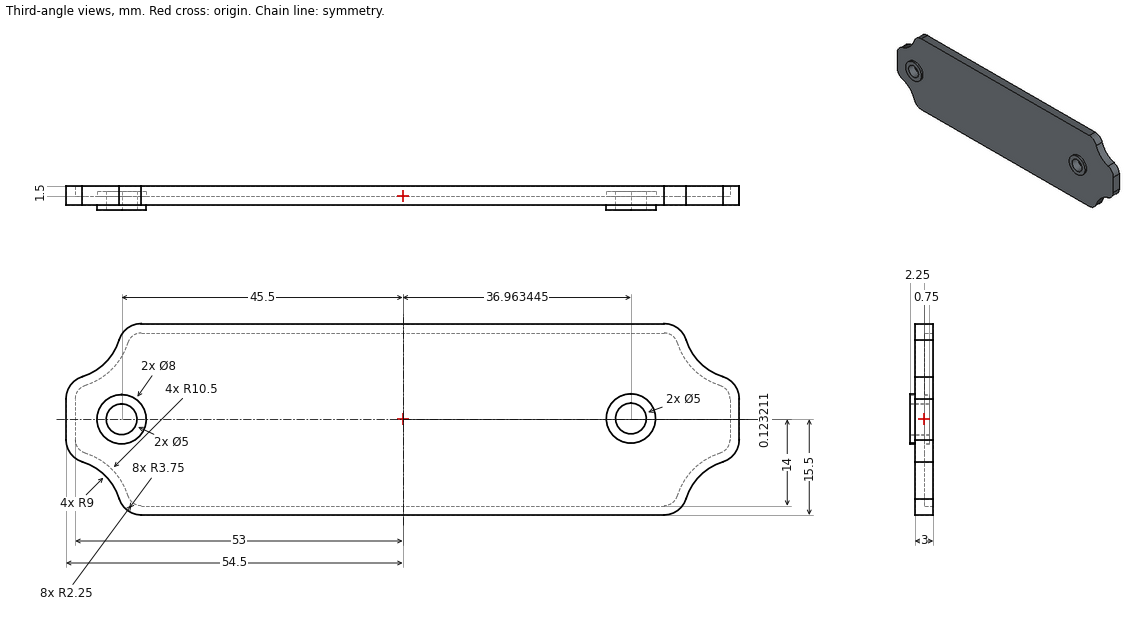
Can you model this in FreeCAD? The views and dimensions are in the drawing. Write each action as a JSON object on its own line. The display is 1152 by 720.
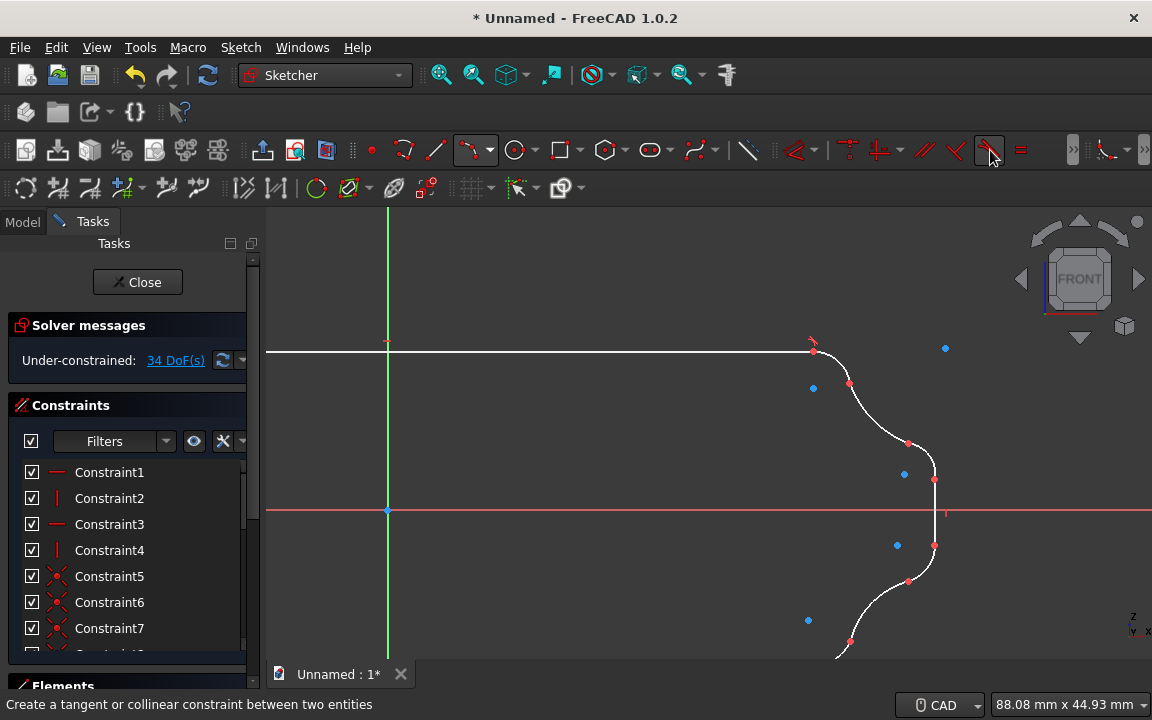
{"action": "scroll", "coordinate": [935, 499], "scroll_direction": "up", "scroll_amount": 2}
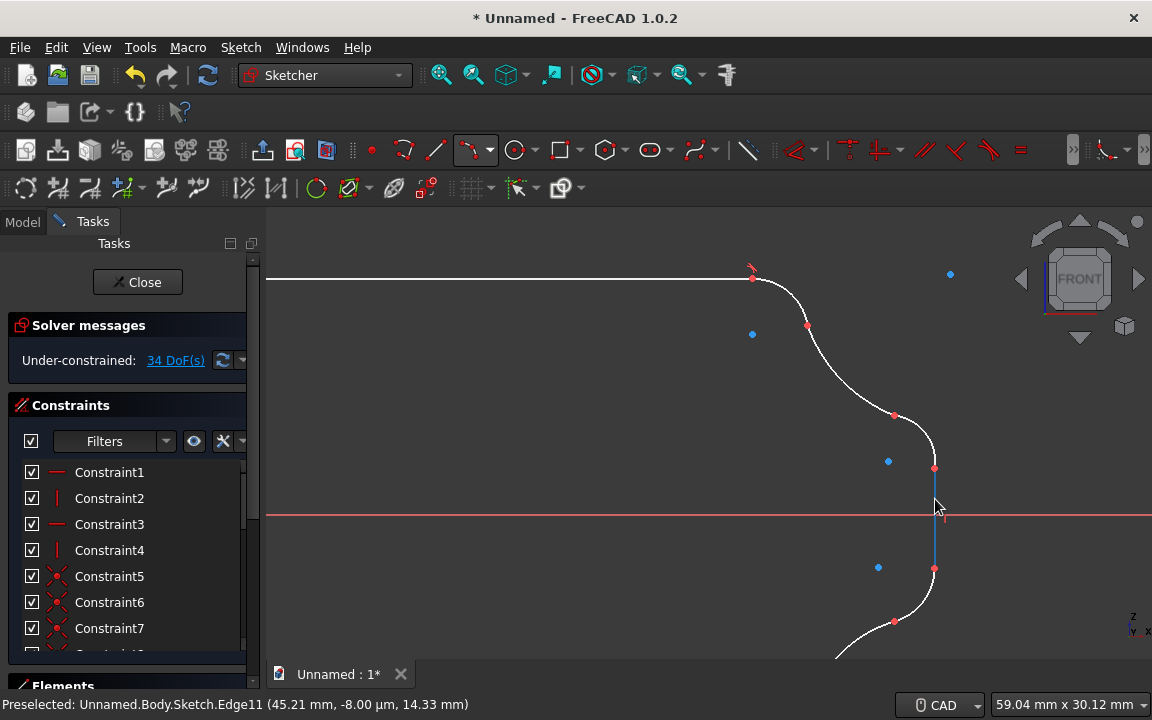
{"action": "left_click", "coordinate": [935, 499]}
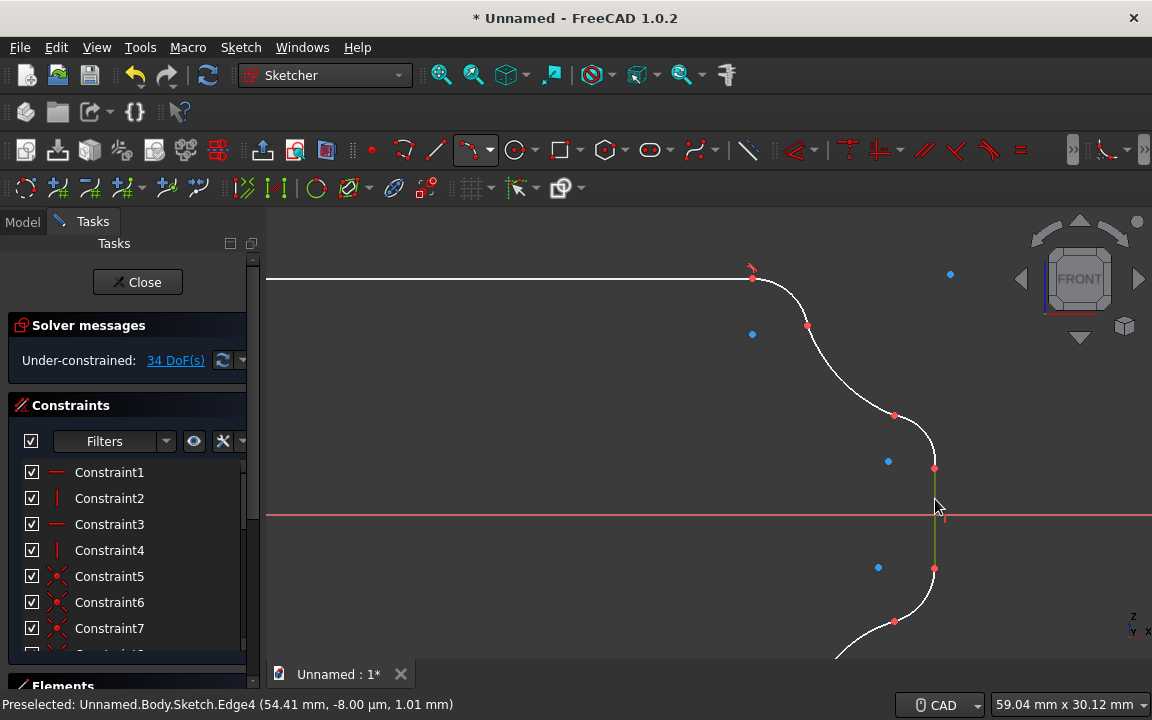
{"action": "left_click", "coordinate": [933, 447]}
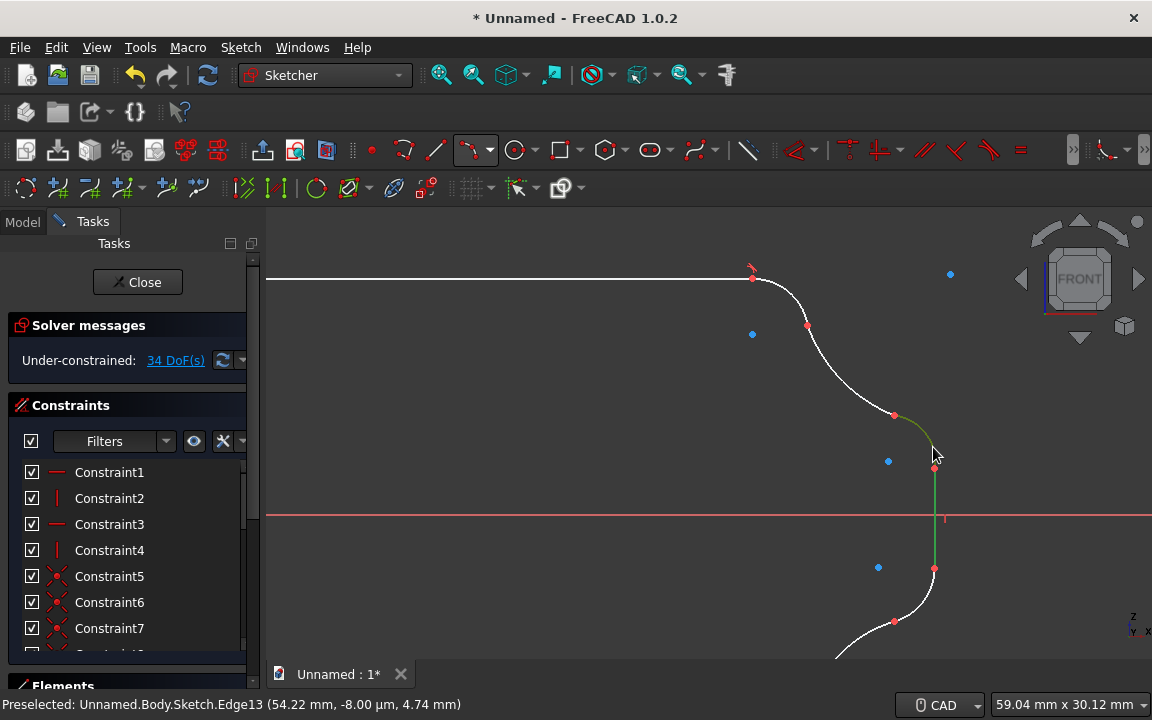
{"action": "left_click", "coordinate": [990, 150]}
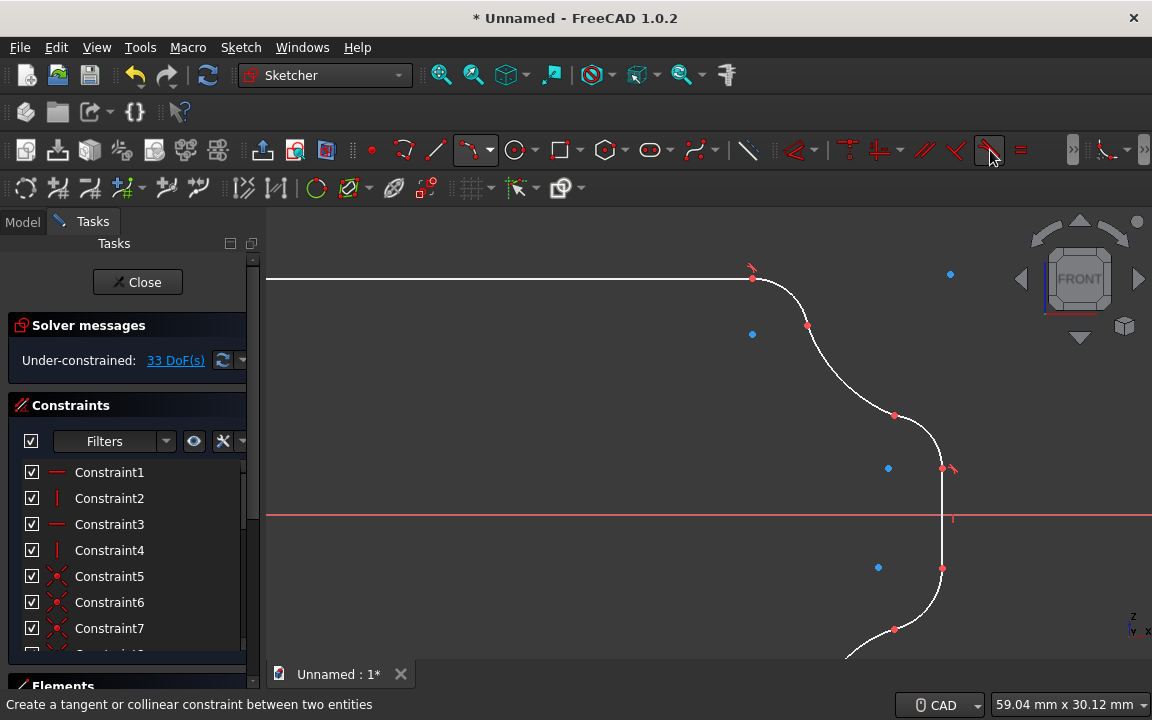
{"action": "left_click", "coordinate": [942, 498]}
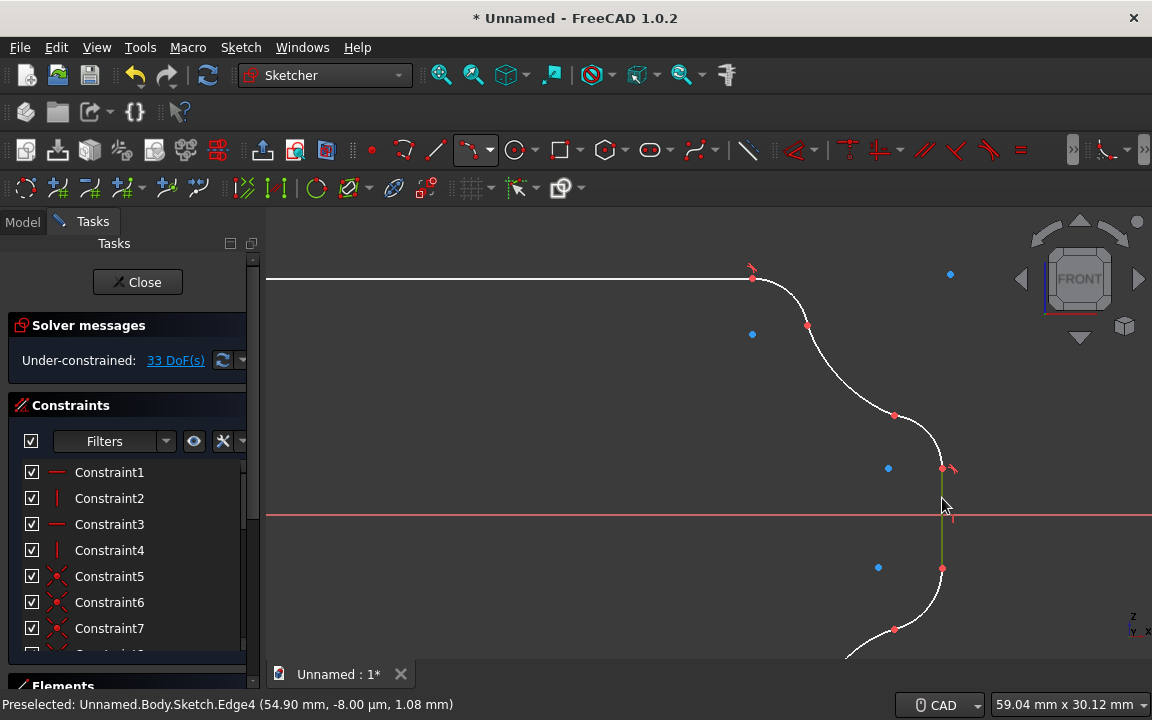
{"action": "left_click", "coordinate": [917, 618]}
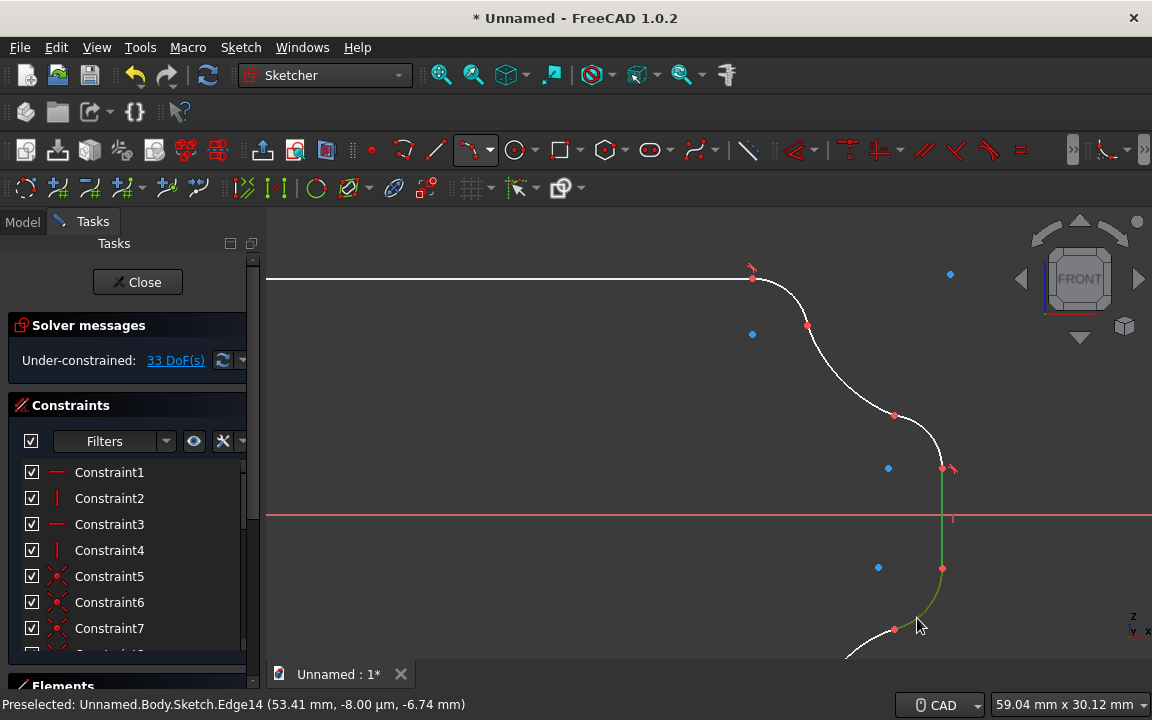
{"action": "left_click", "coordinate": [990, 150]}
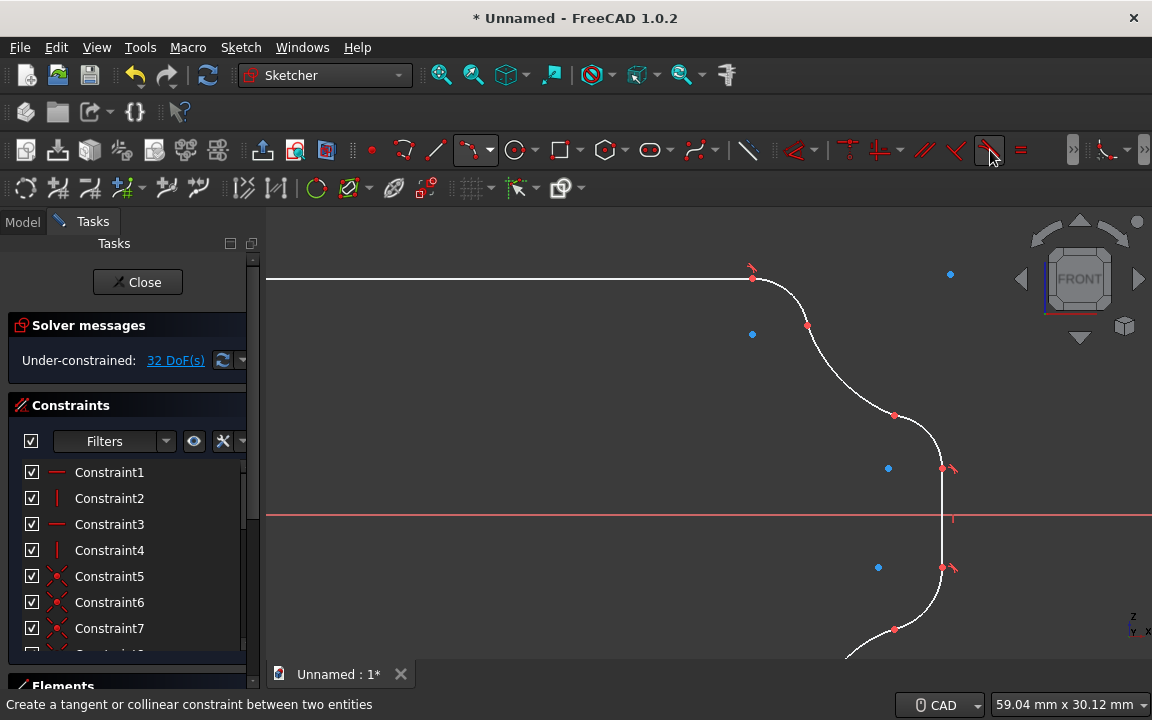
{"action": "scroll", "coordinate": [866, 398], "scroll_direction": "down", "scroll_amount": 6}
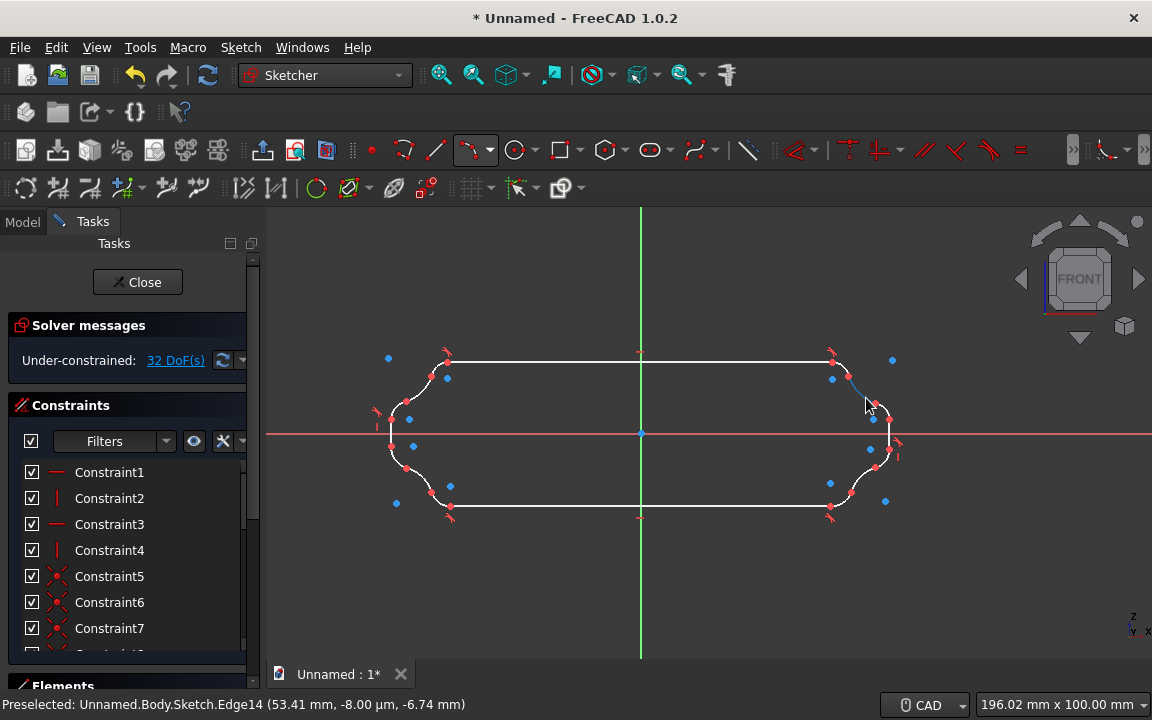
{"action": "scroll", "coordinate": [435, 499], "scroll_direction": "up", "scroll_amount": 4}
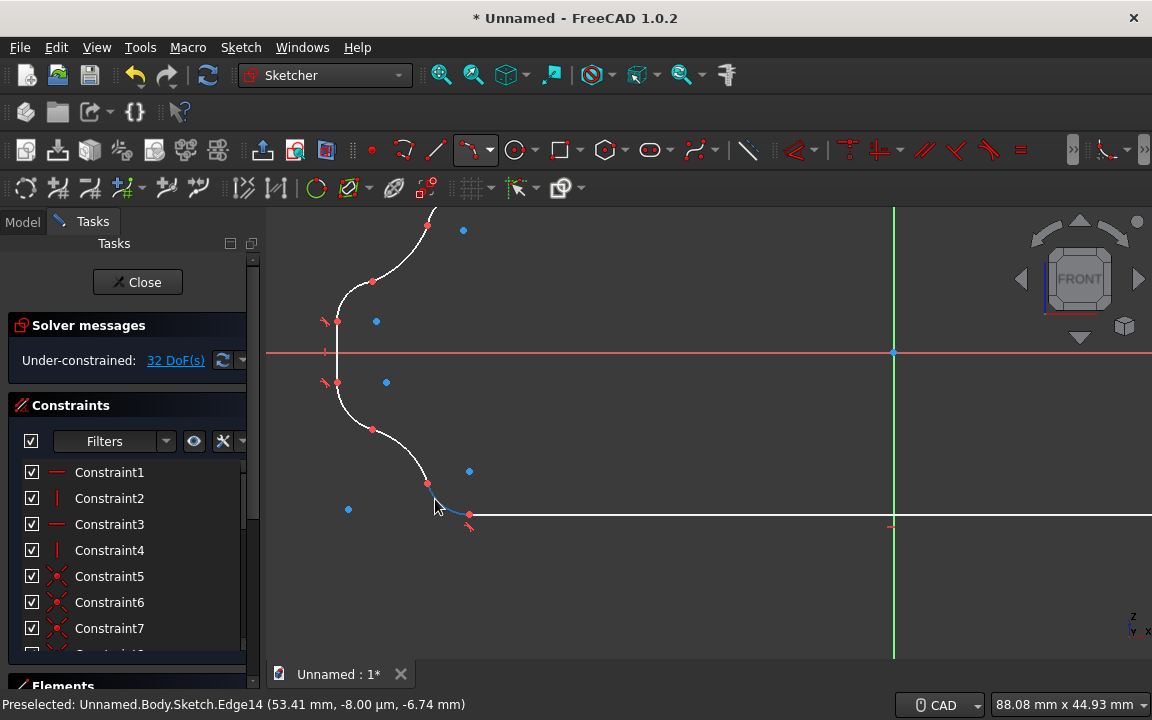
{"action": "left_click", "coordinate": [436, 499]}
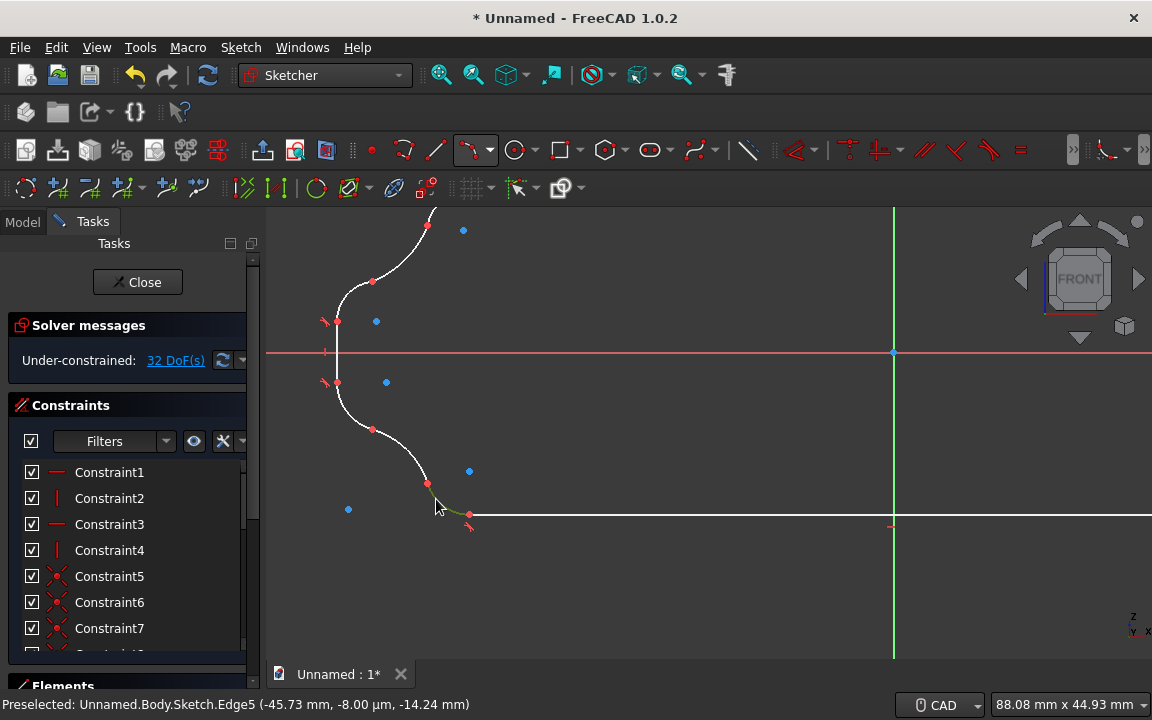
{"action": "left_click", "coordinate": [417, 462]}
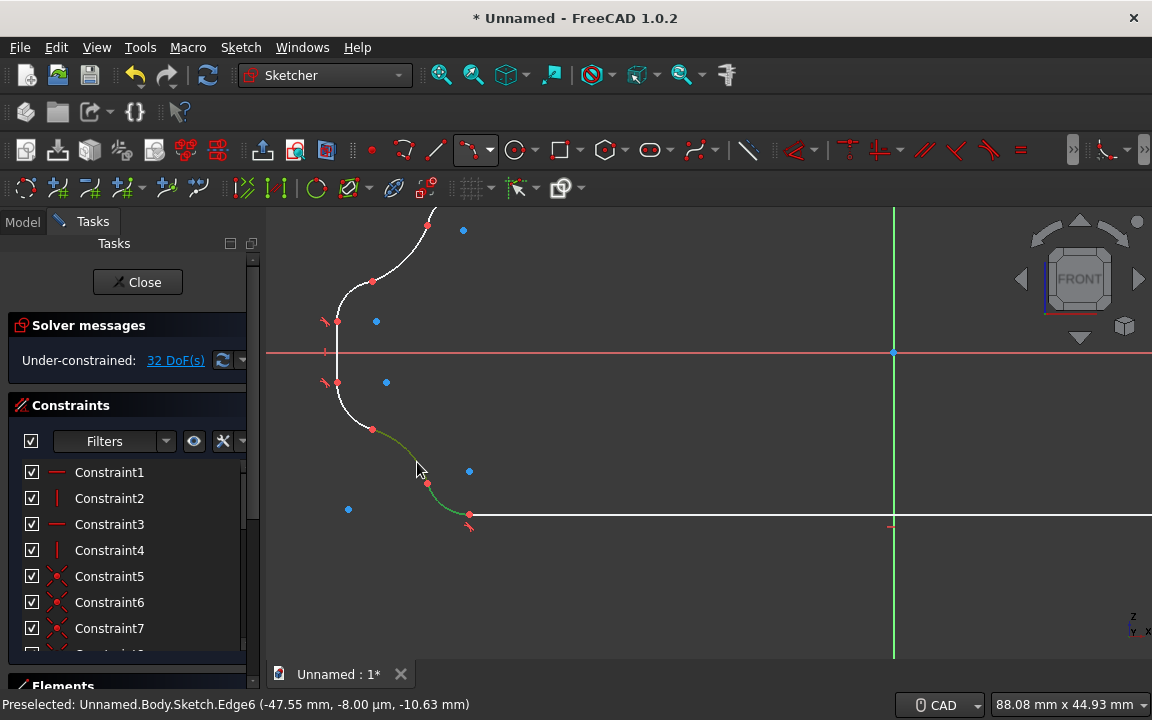
{"action": "left_click", "coordinate": [990, 150]}